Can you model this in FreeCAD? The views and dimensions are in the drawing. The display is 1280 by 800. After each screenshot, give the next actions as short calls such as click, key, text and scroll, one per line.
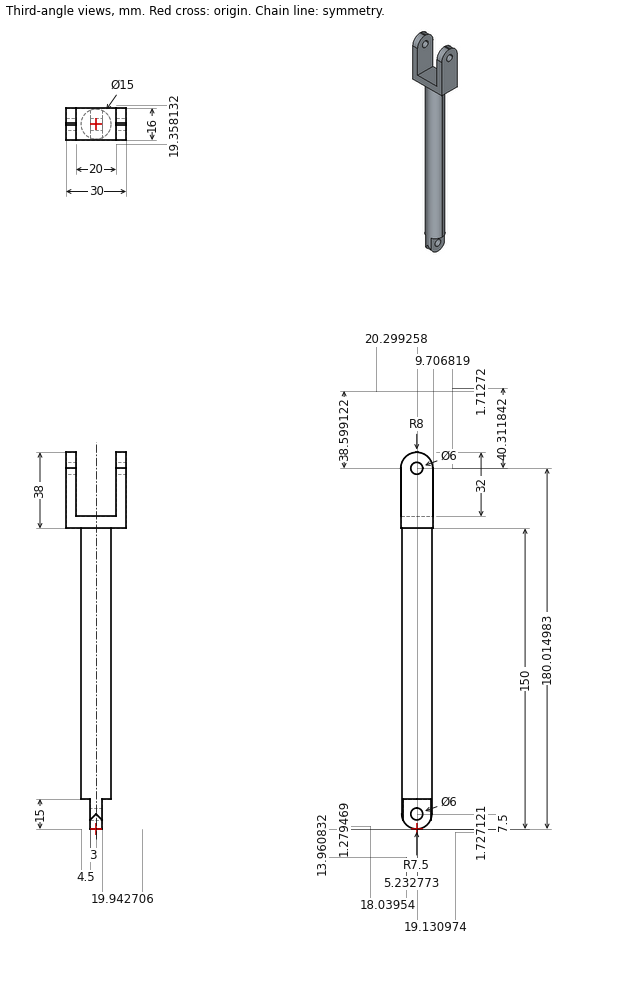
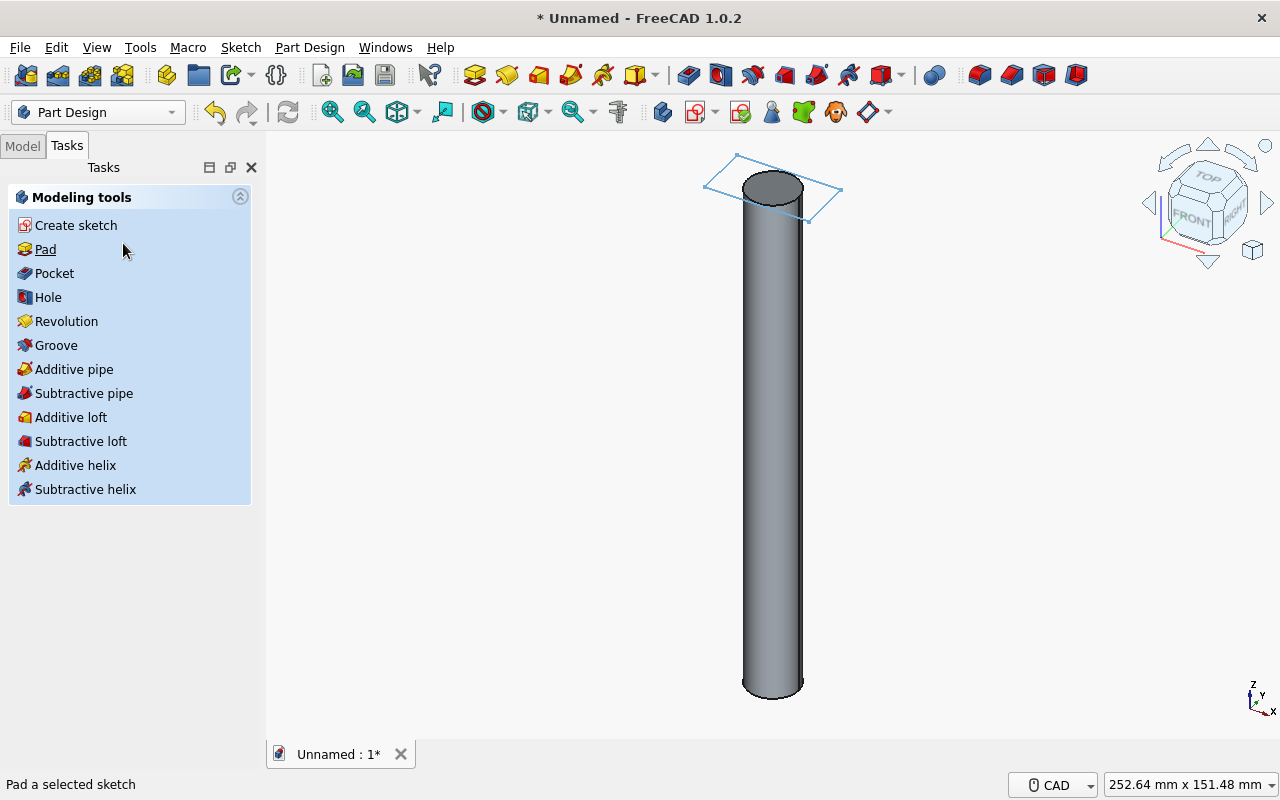
click(476, 76)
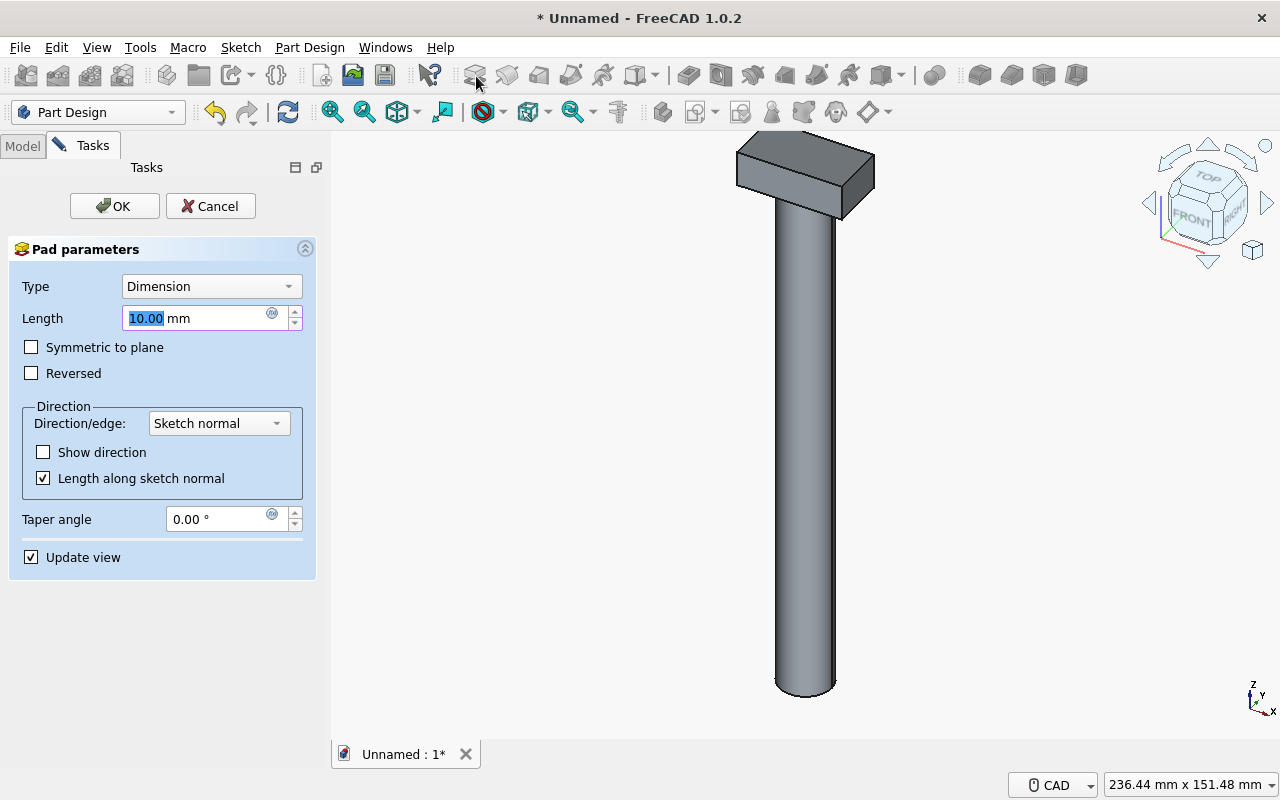
text(38)
key(Tab)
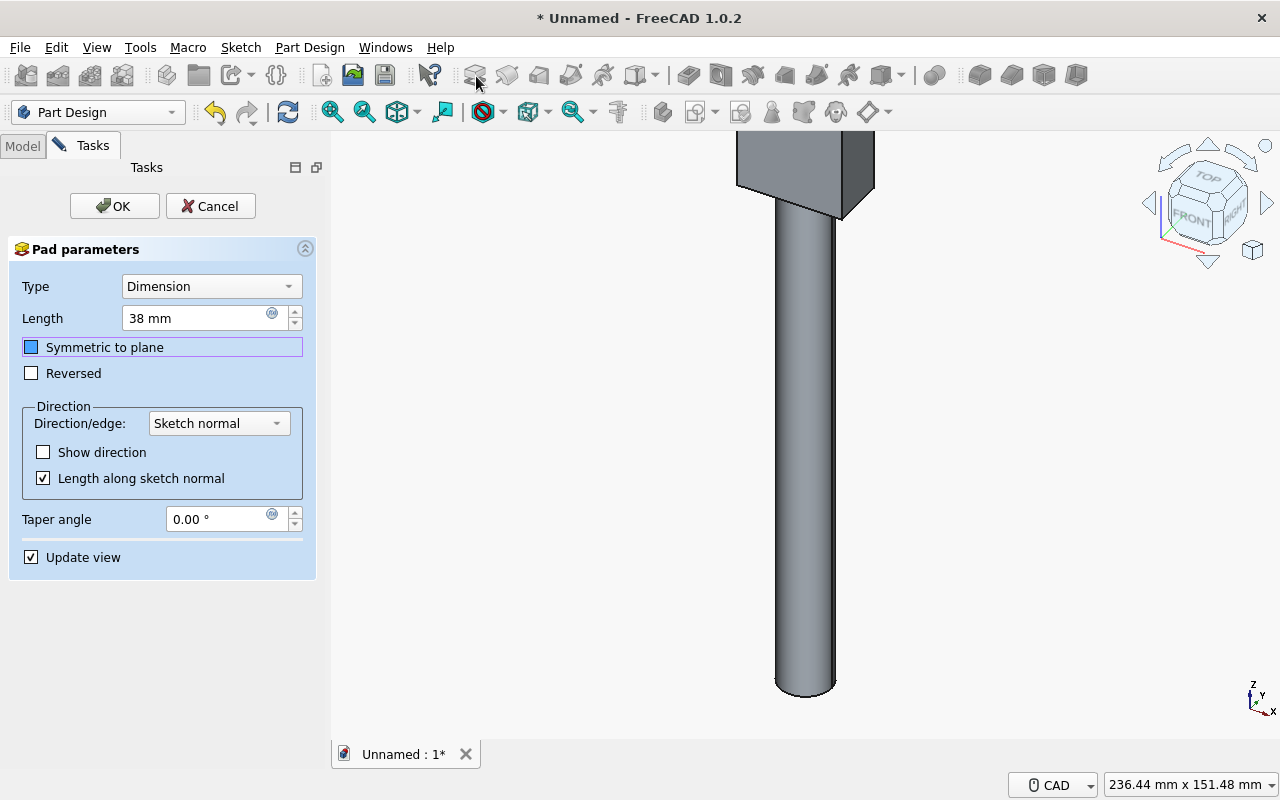
click(115, 206)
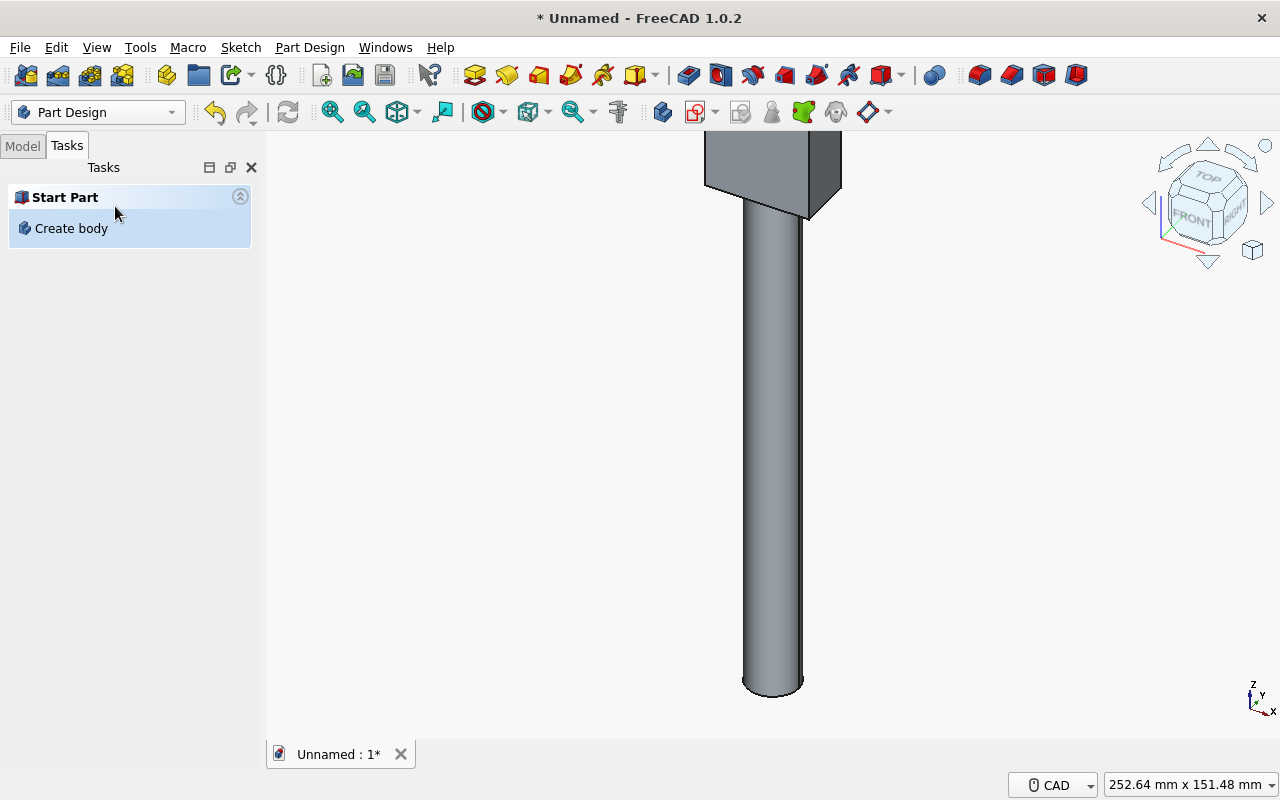
key(v)
key(f)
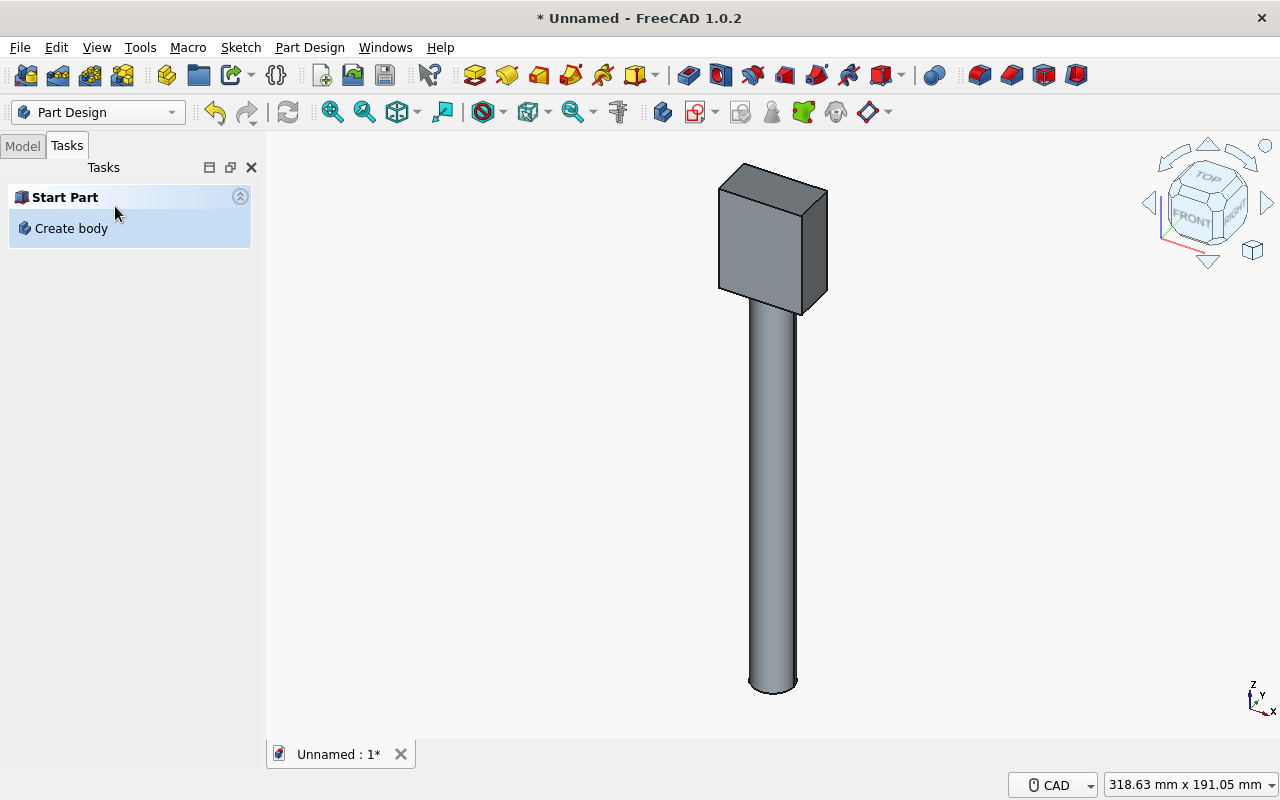
click(785, 193)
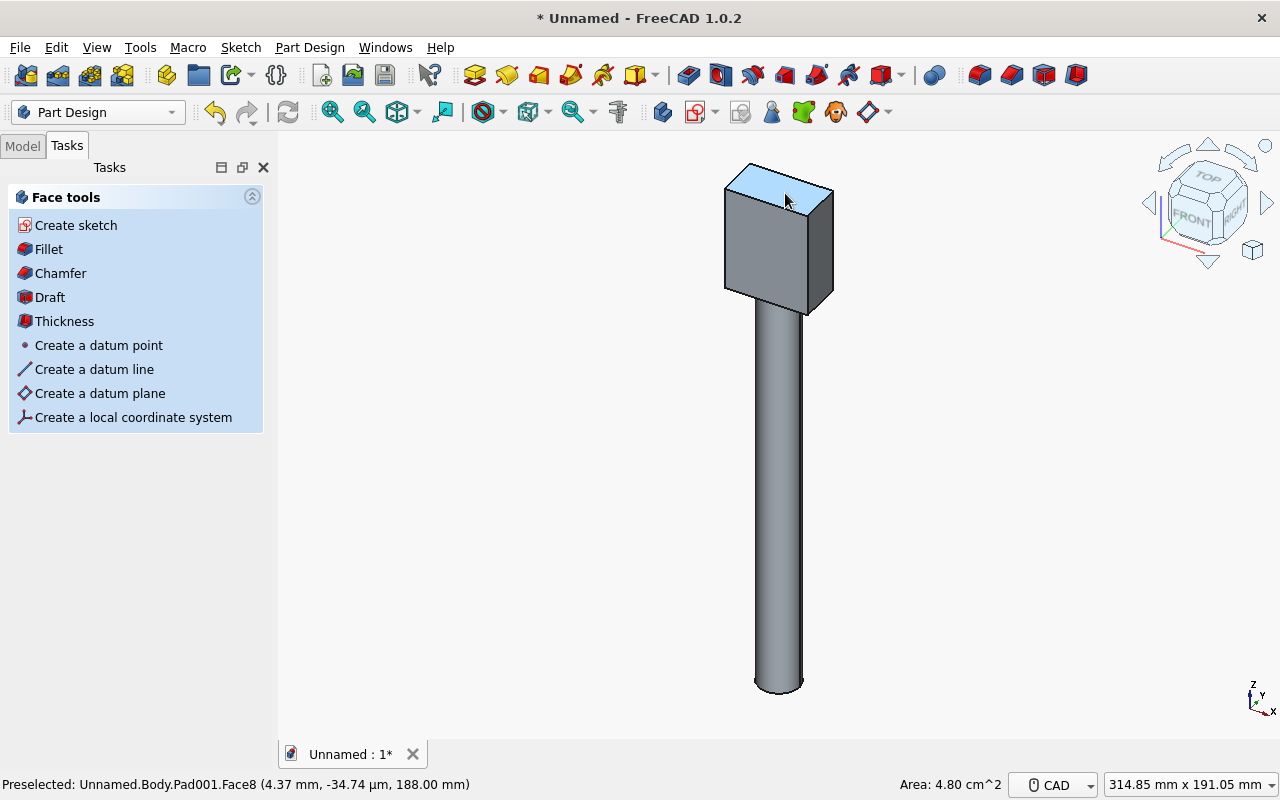
click(696, 112)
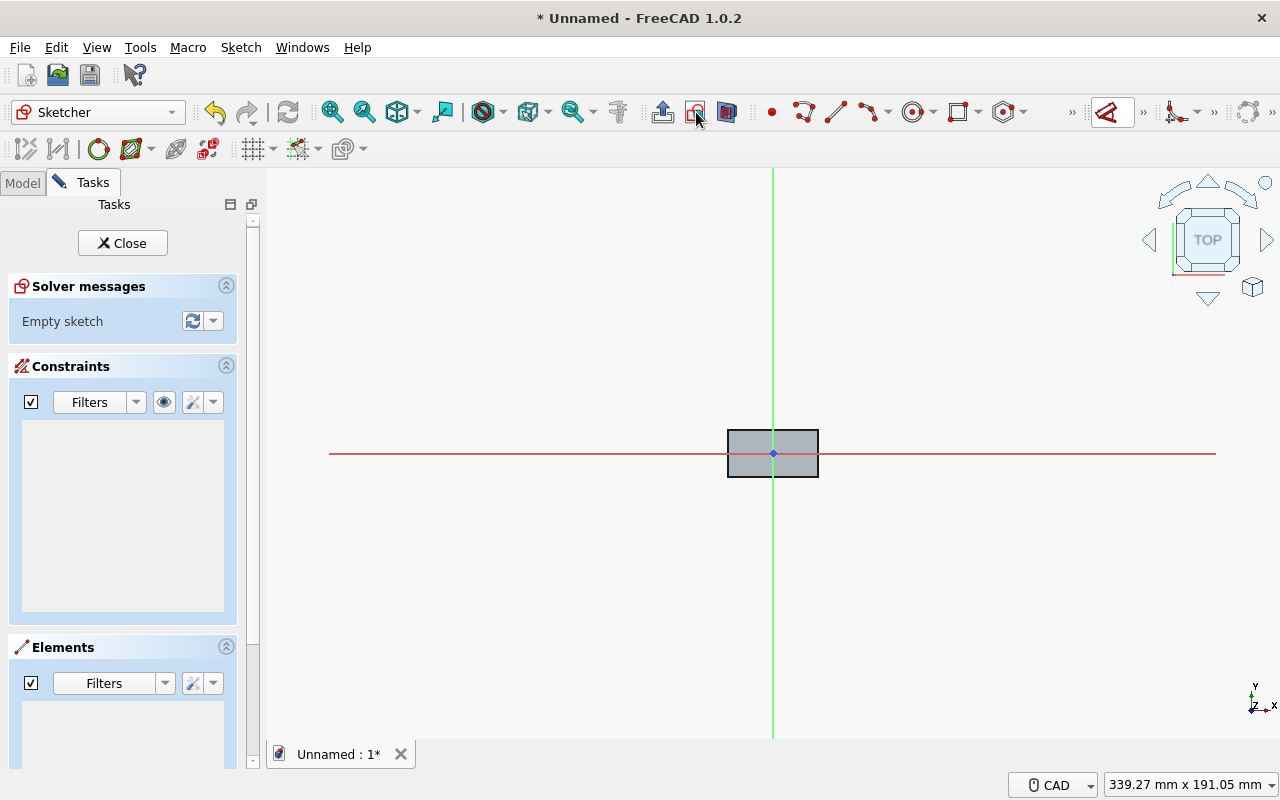
scroll(787, 454, up, 9)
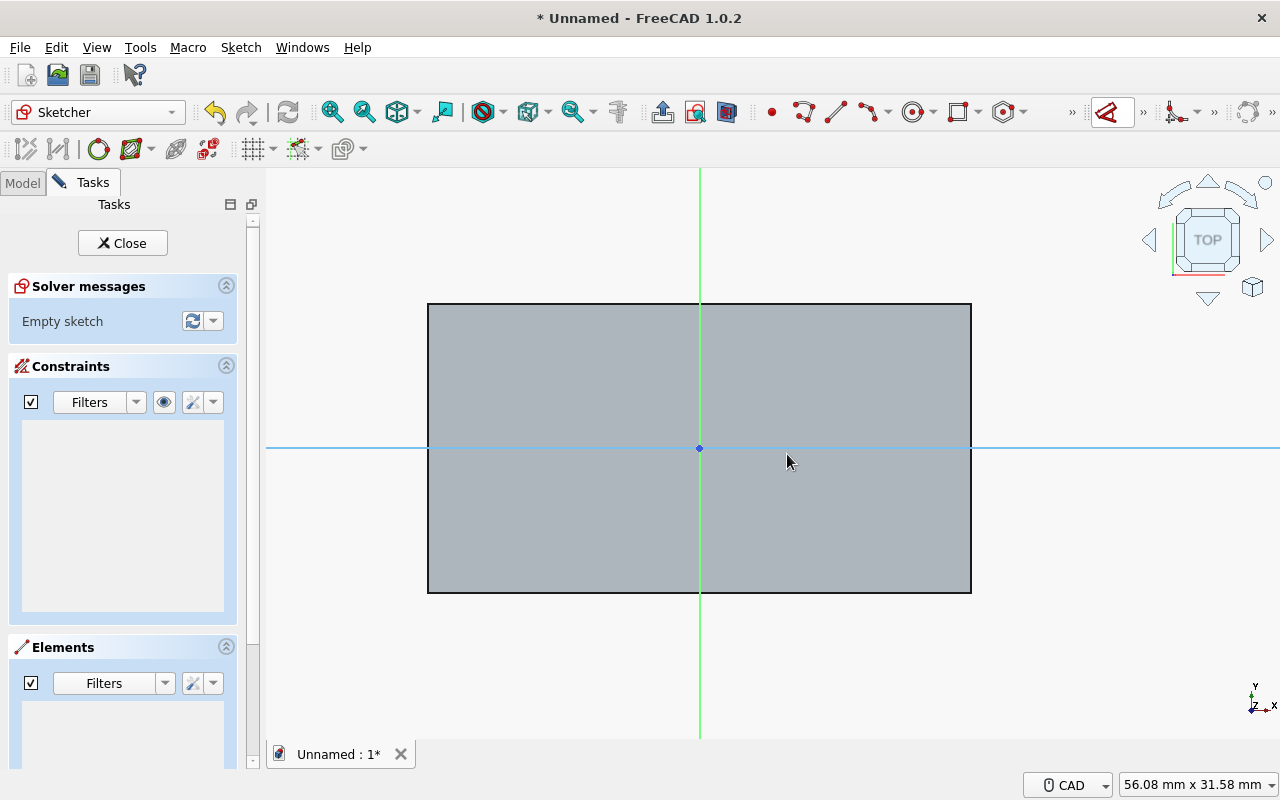
key(g)
key(v)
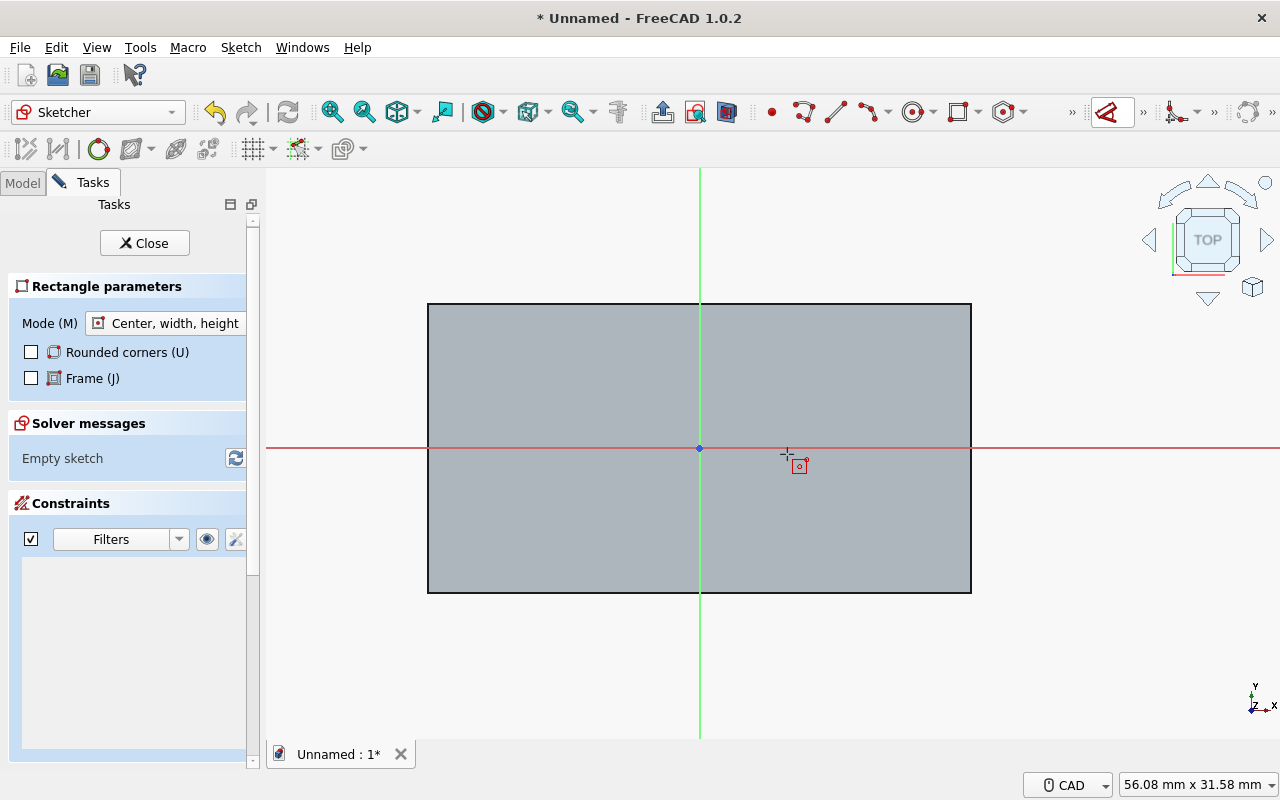
click(700, 448)
move(881, 273)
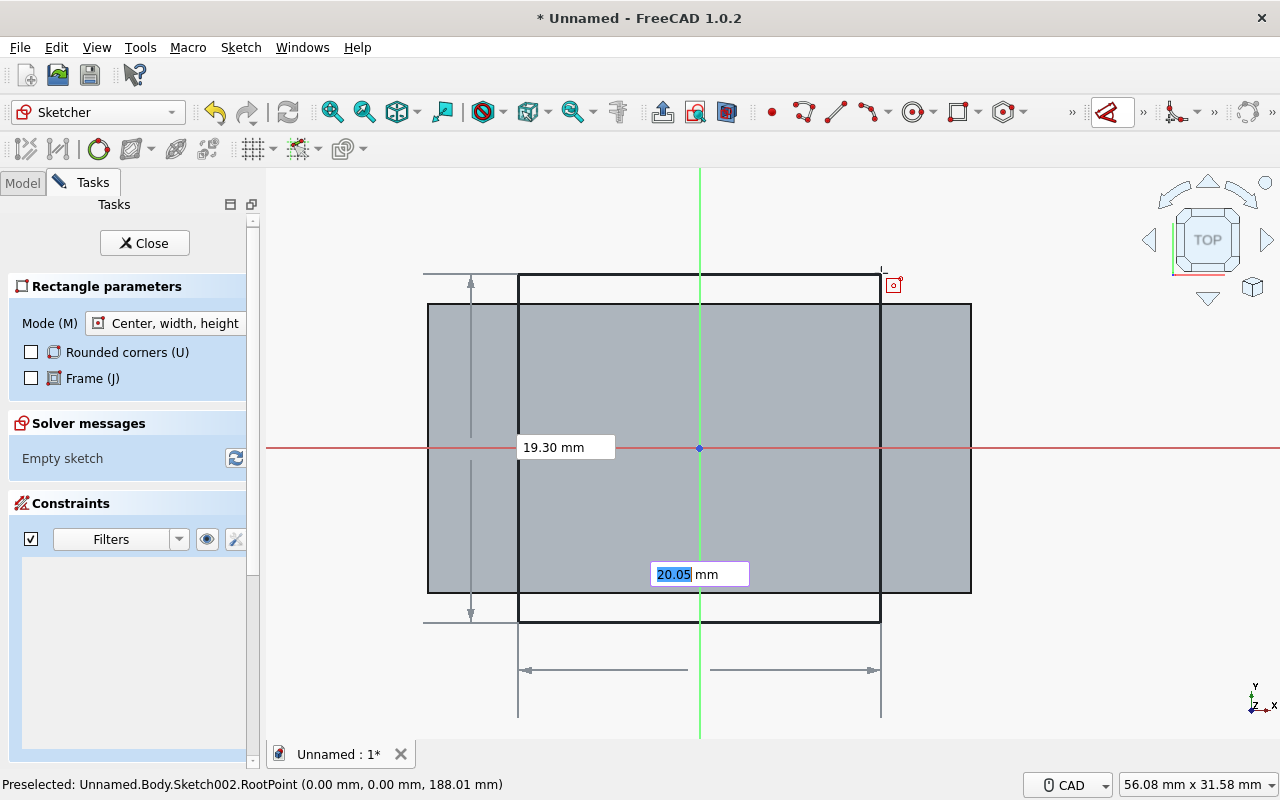
text(20)
key(Tab)
text(19.358132)
key(Return)
key(Escape)